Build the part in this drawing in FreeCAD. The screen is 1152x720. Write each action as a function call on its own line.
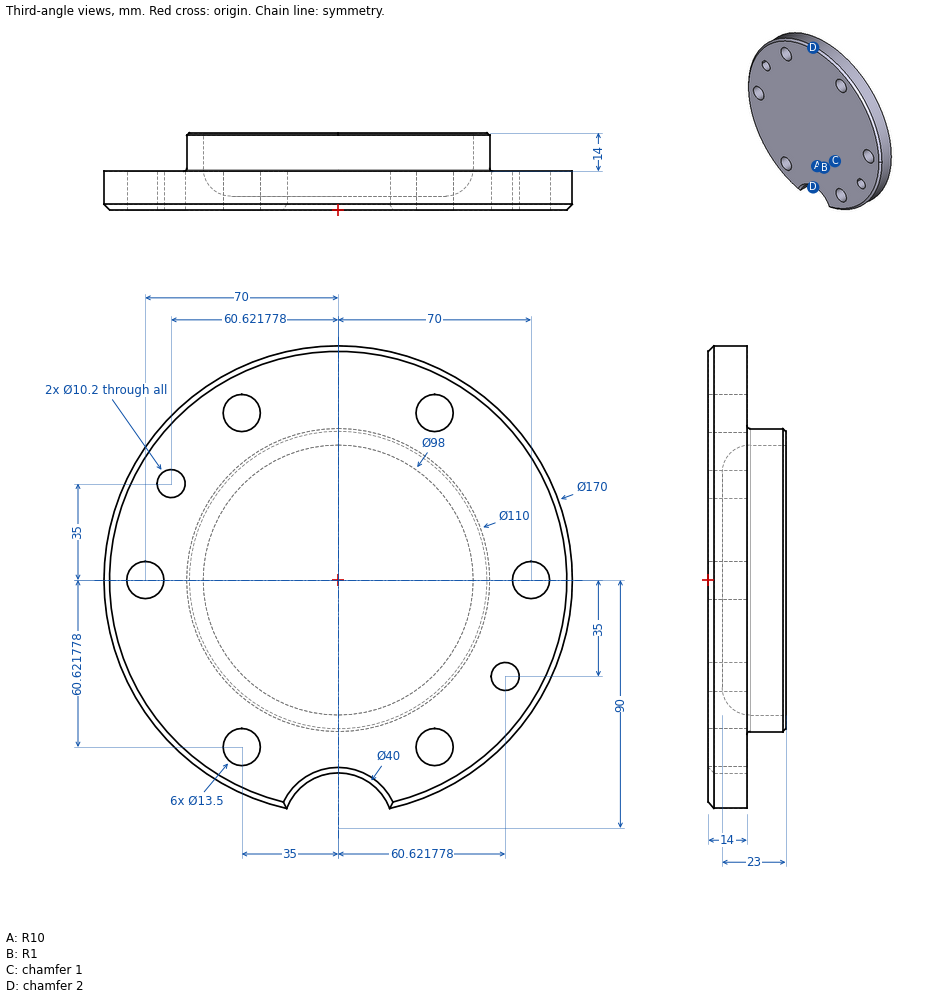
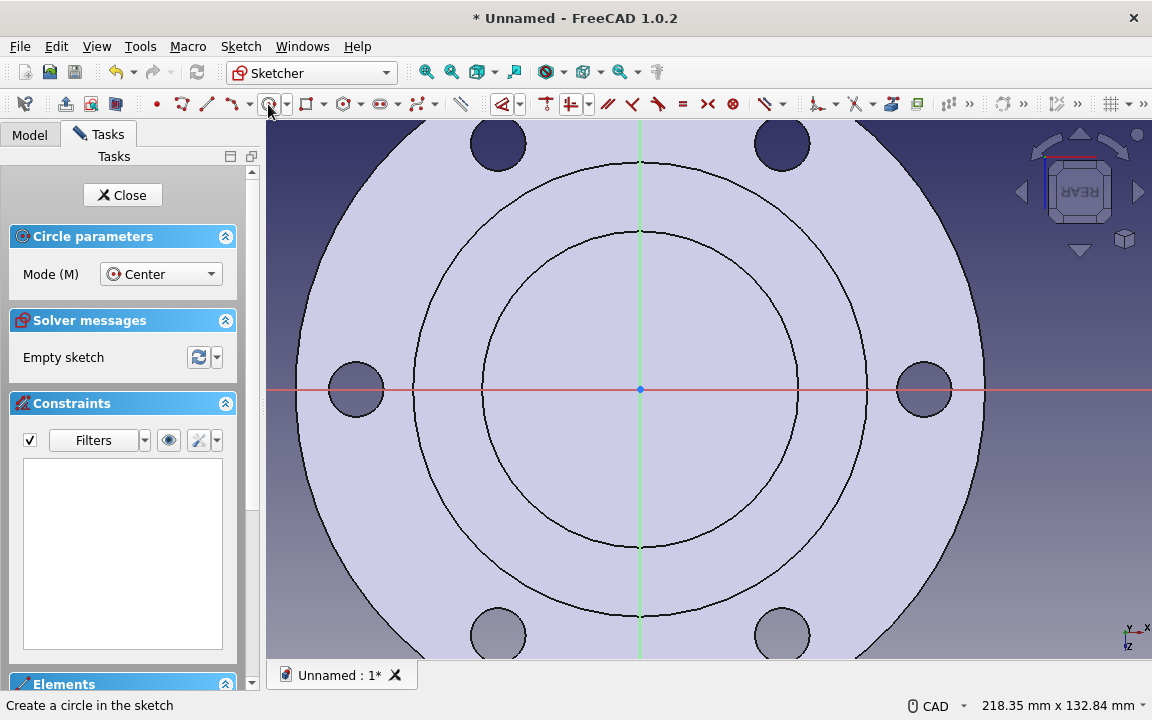
click(394, 532)
click(409, 517)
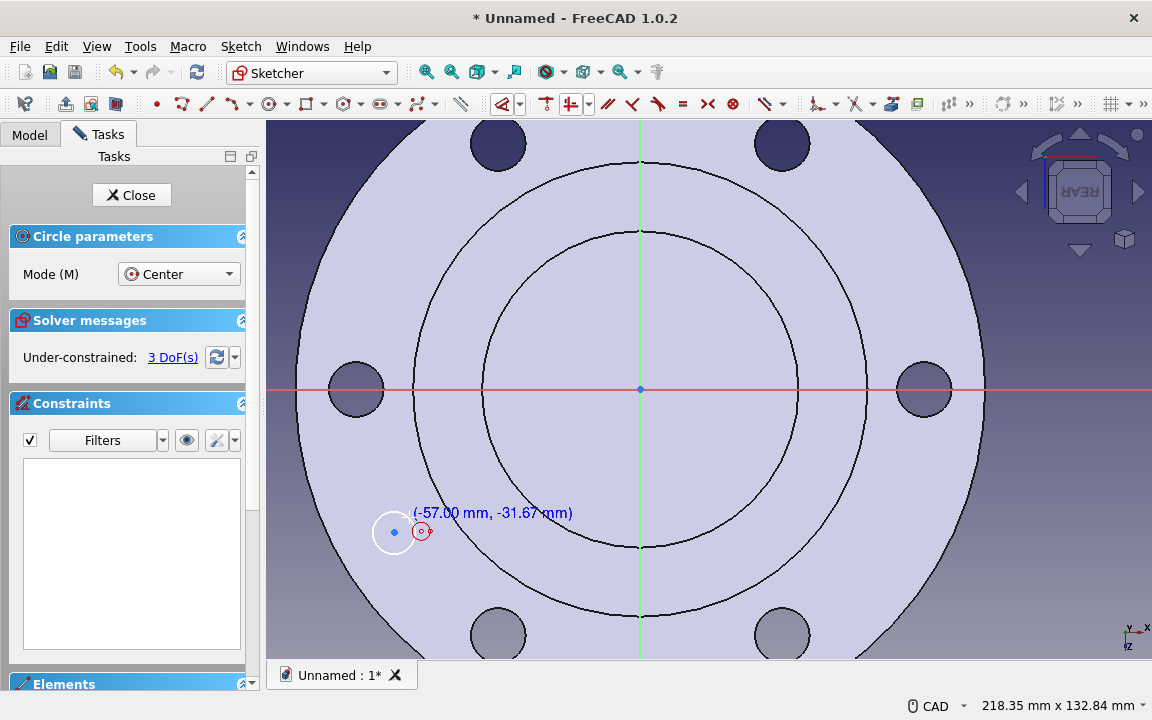
click(886, 247)
click(901, 233)
key(Escape)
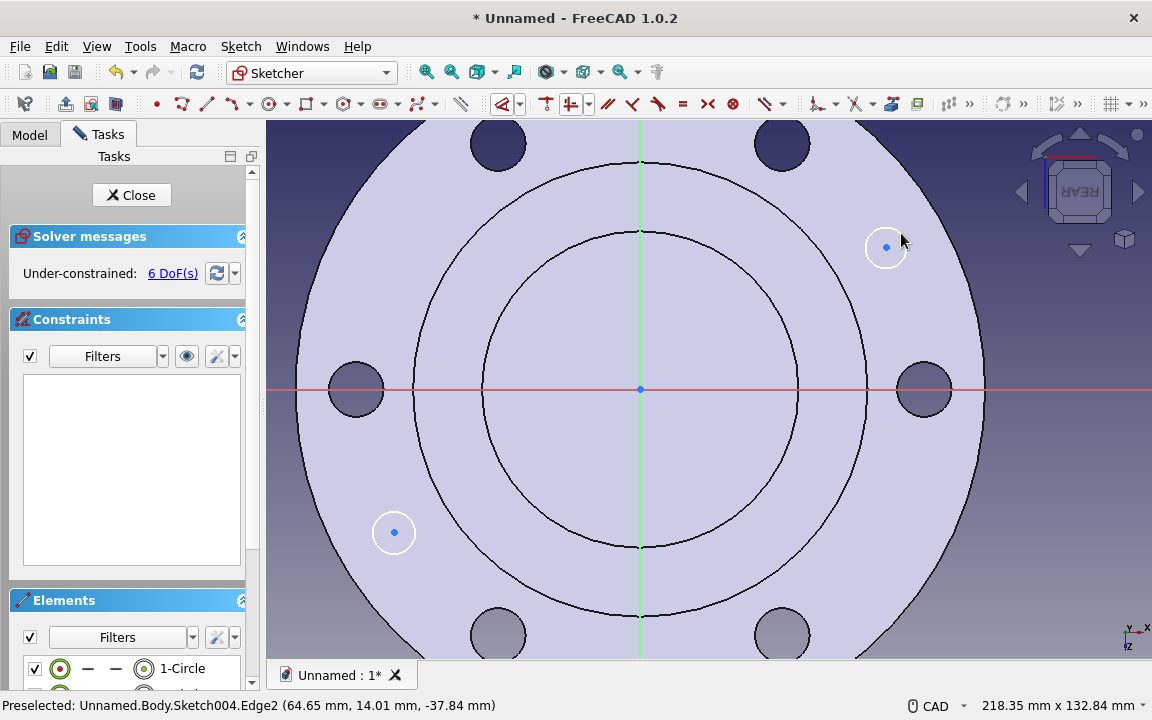
click(409, 518)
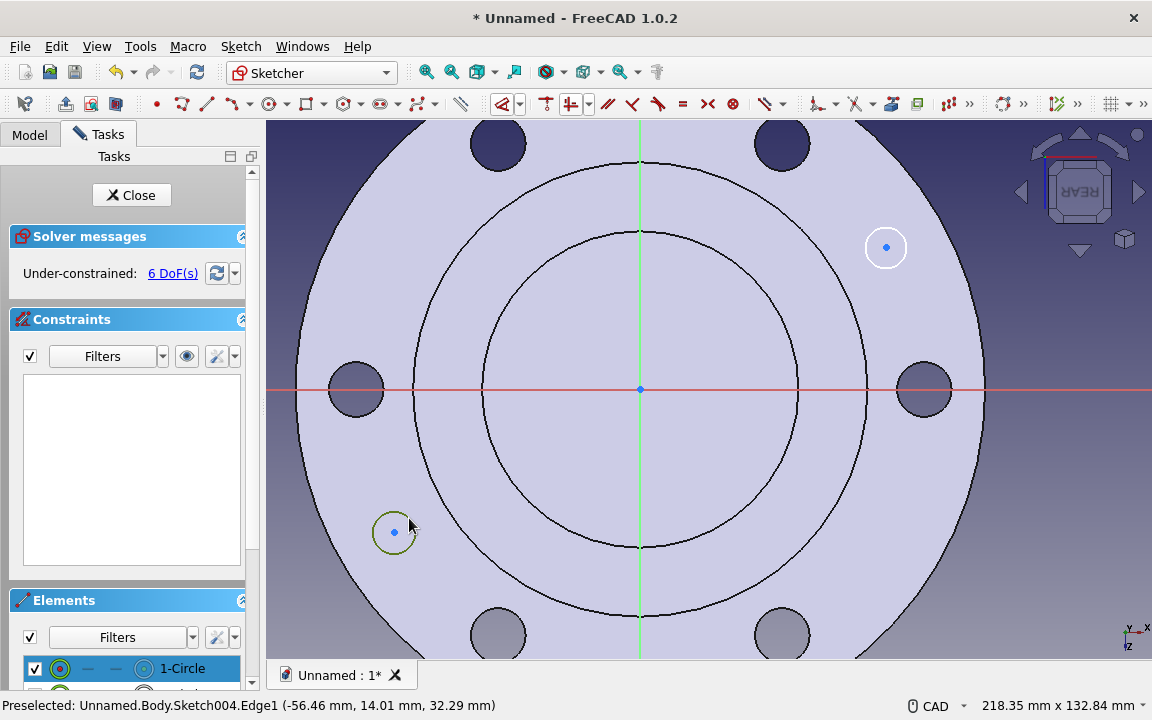
click(900, 233)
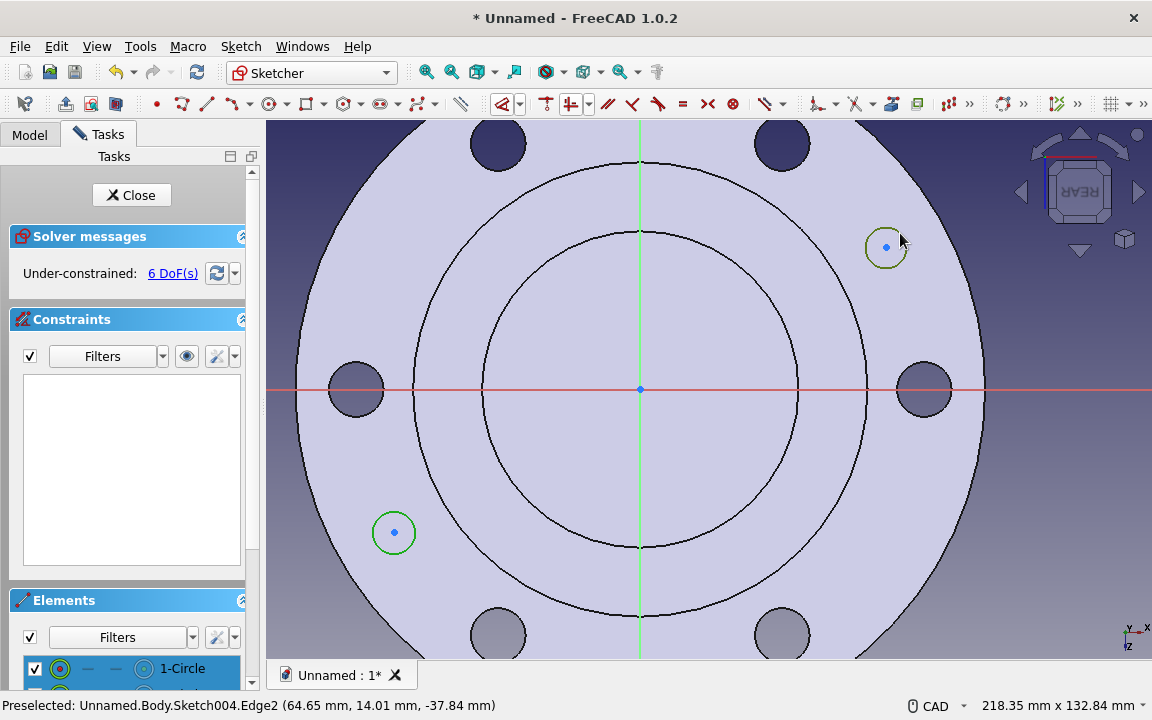
click(683, 104)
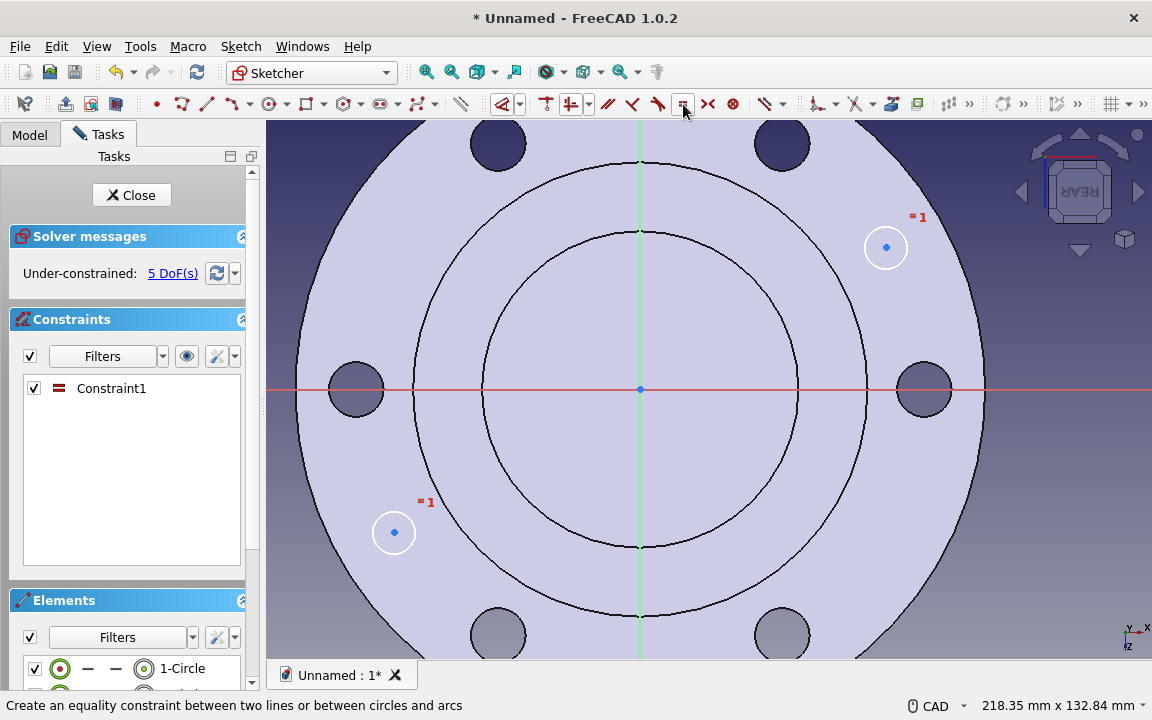
click(409, 518)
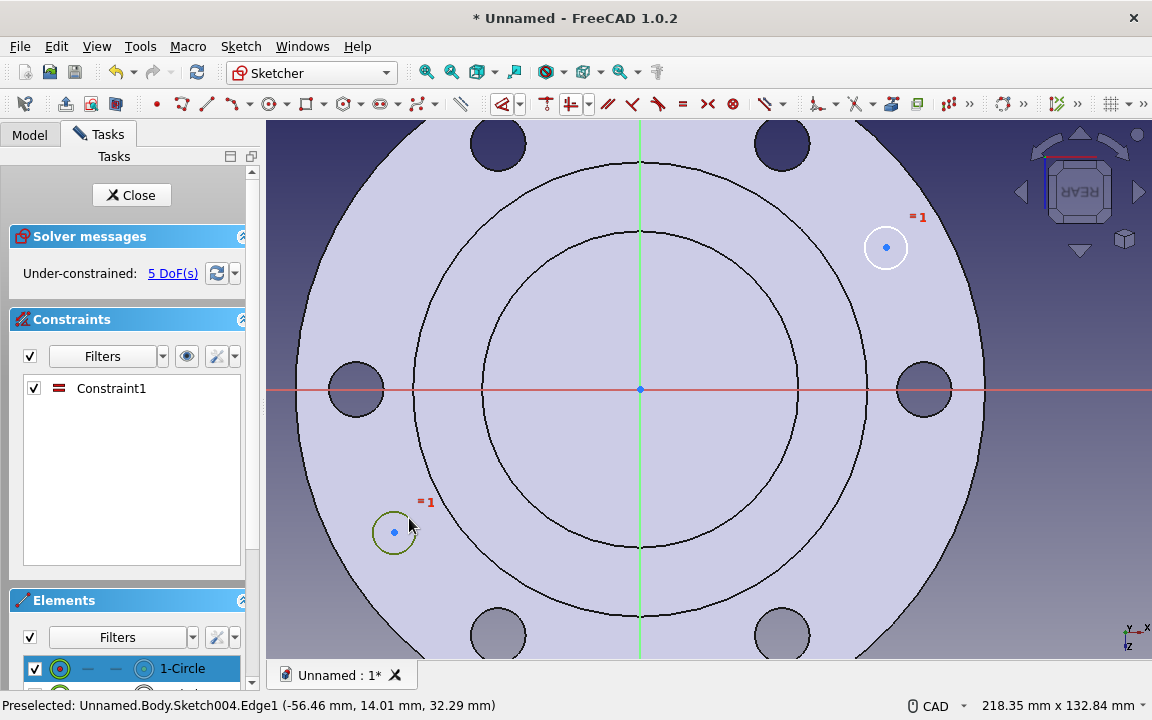
click(520, 104)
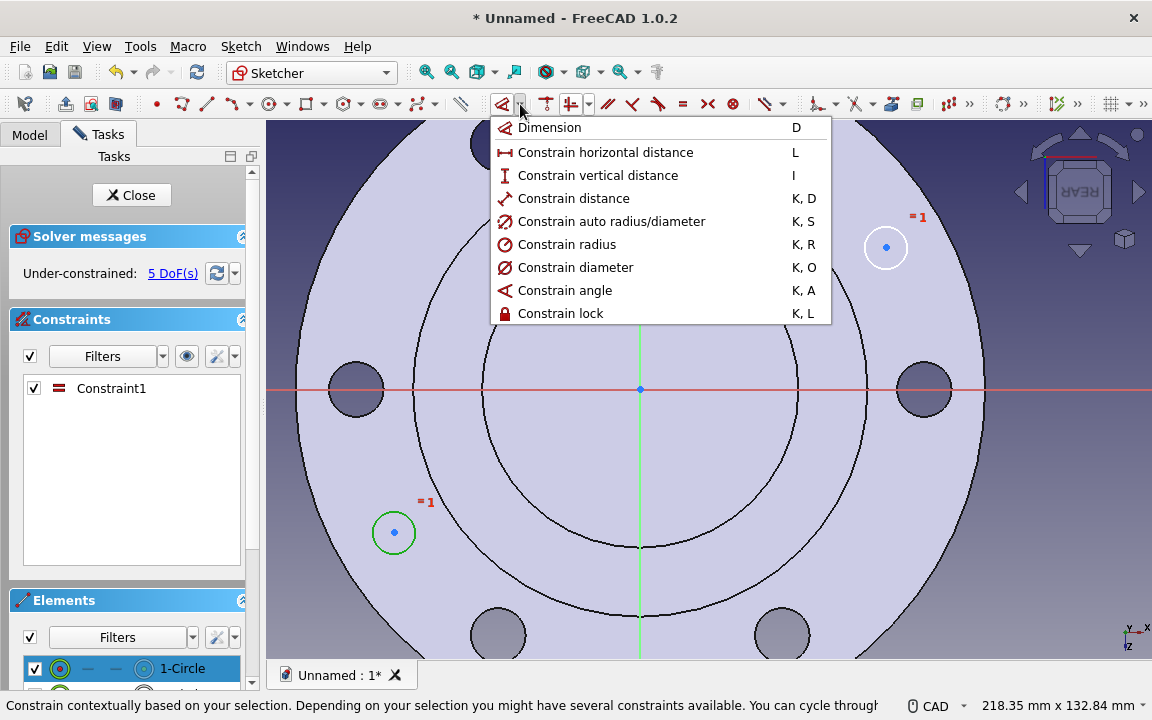
click(661, 268)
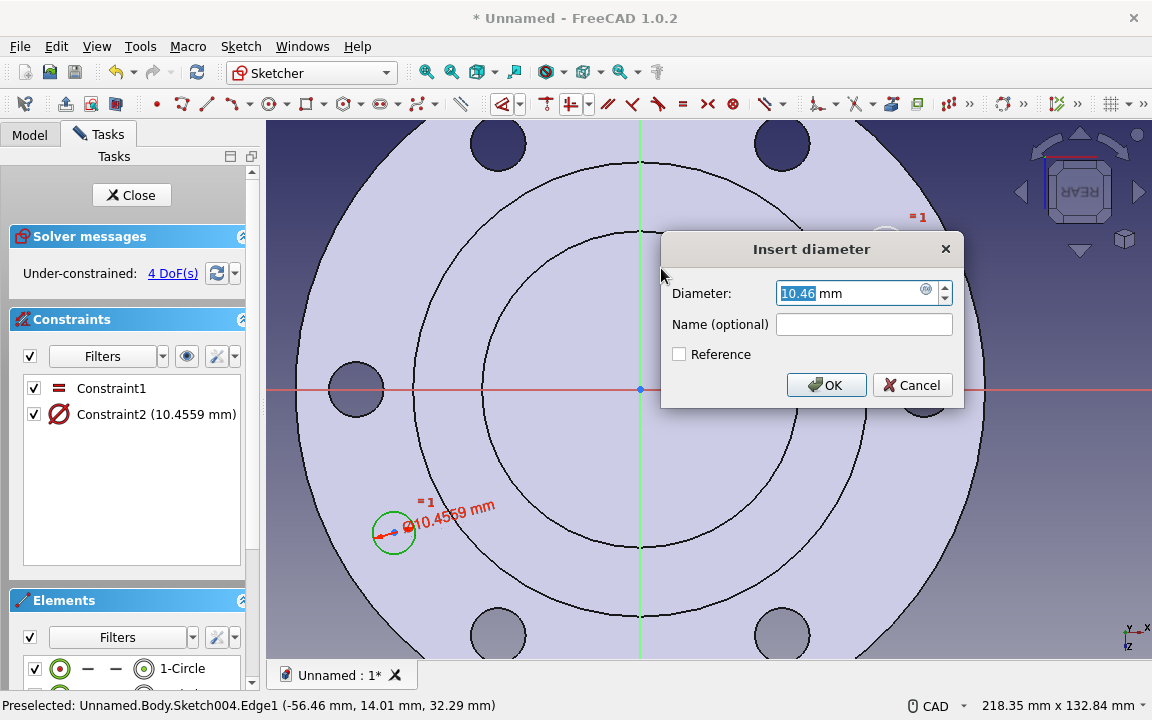
text(10.2)
key(Return)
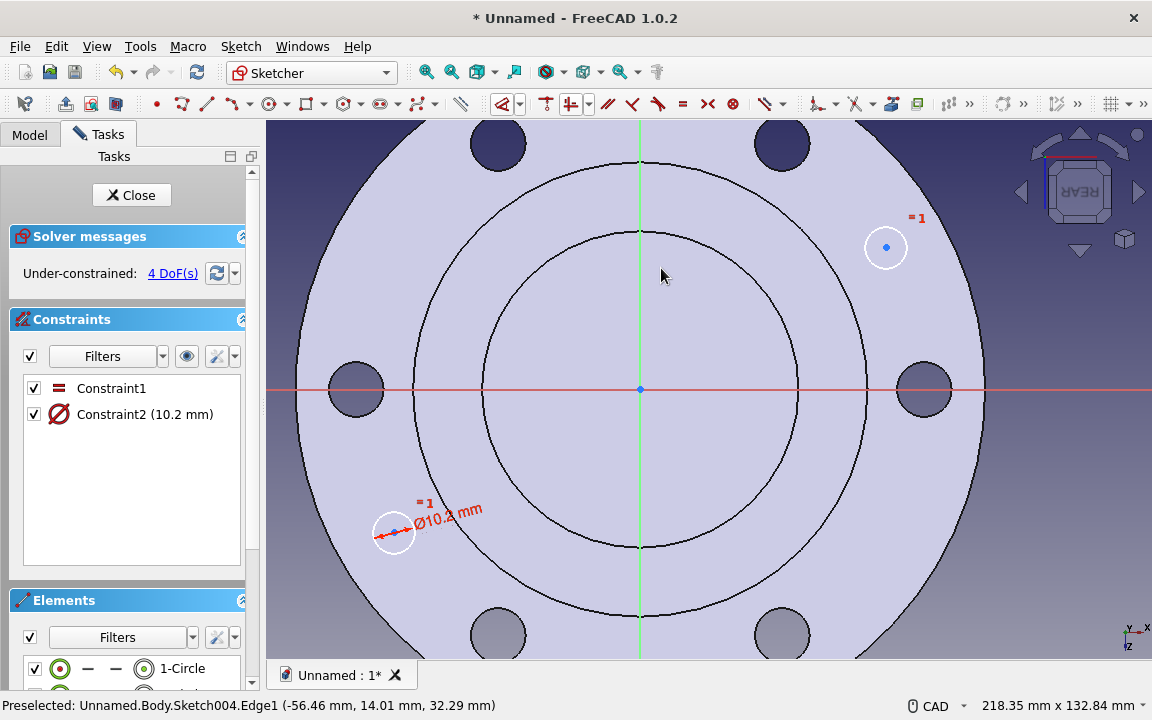
click(394, 533)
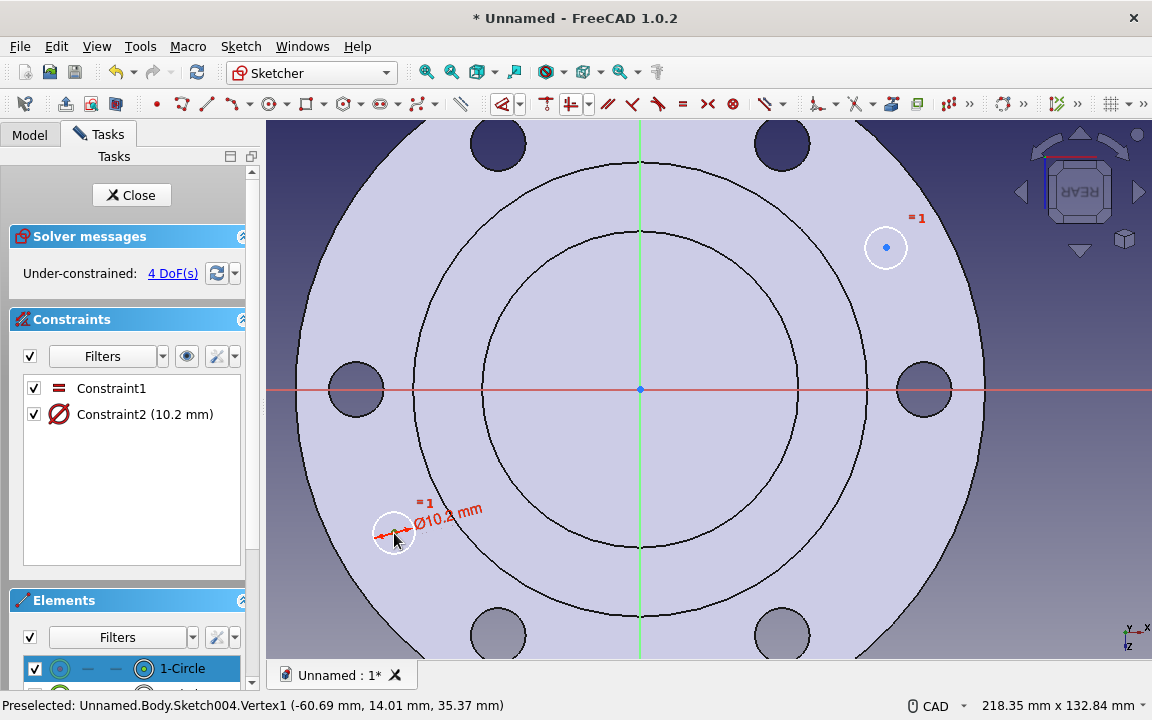
click(520, 104)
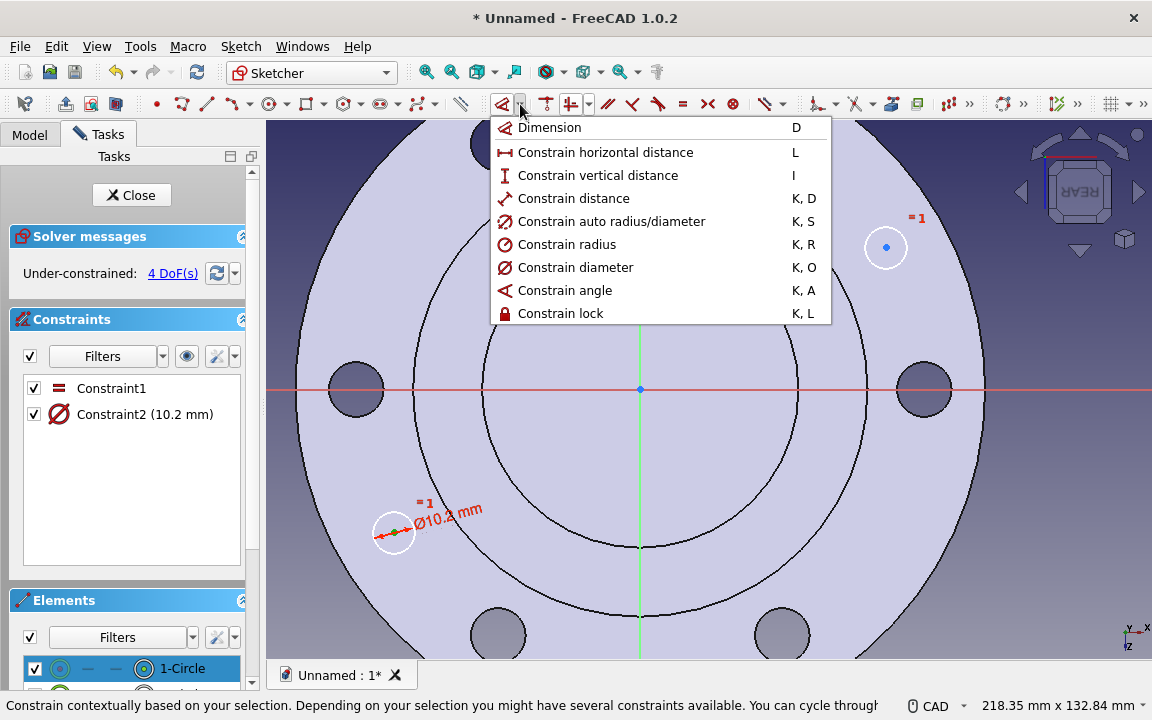
click(661, 176)